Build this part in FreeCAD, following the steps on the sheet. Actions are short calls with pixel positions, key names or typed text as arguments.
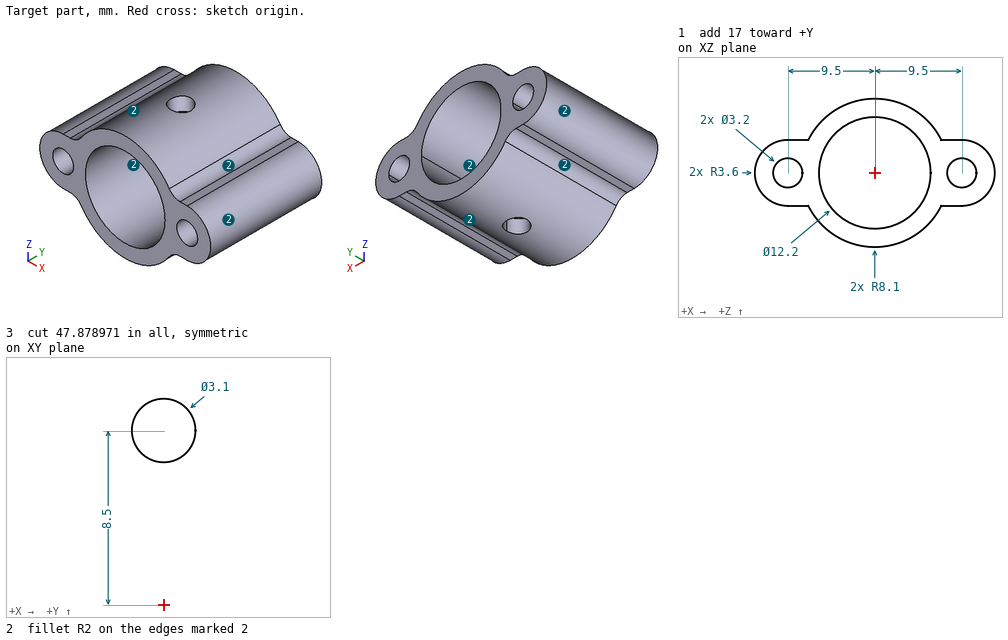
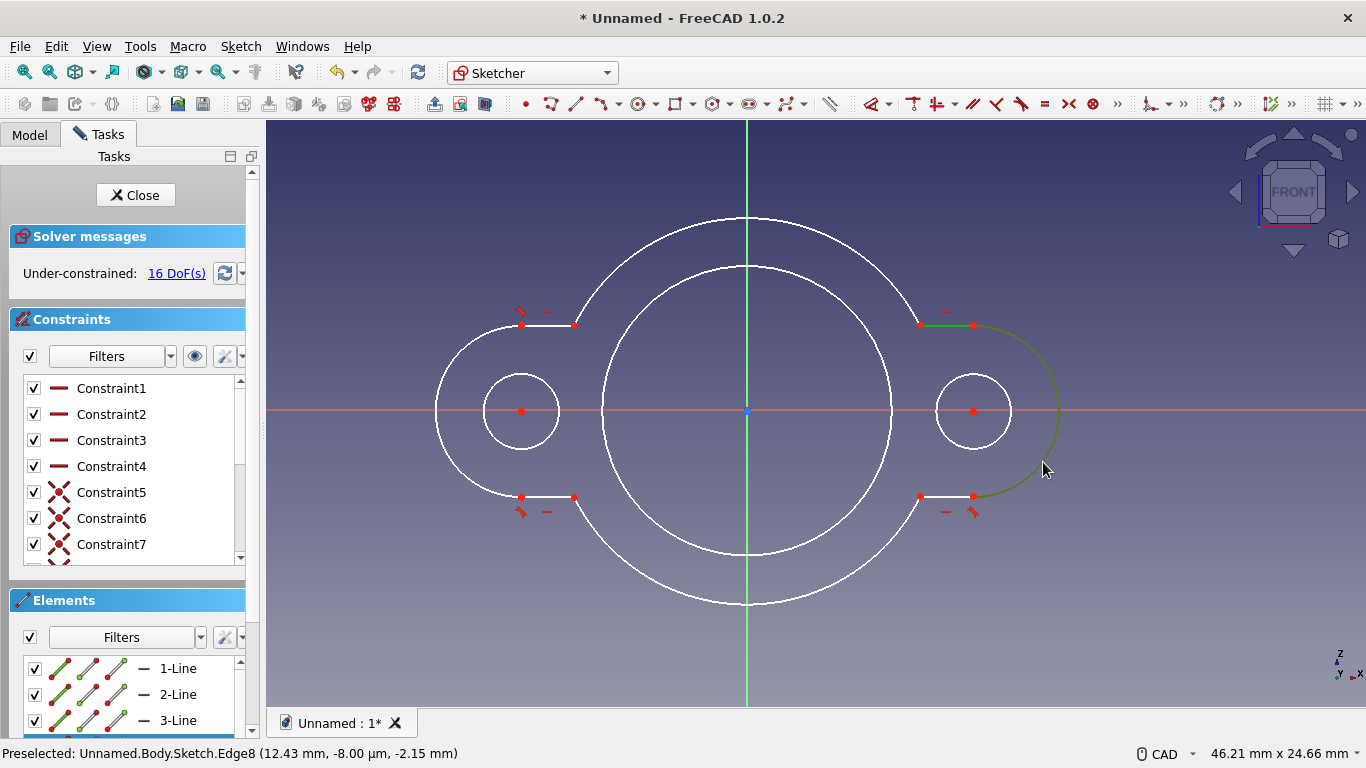
key(t)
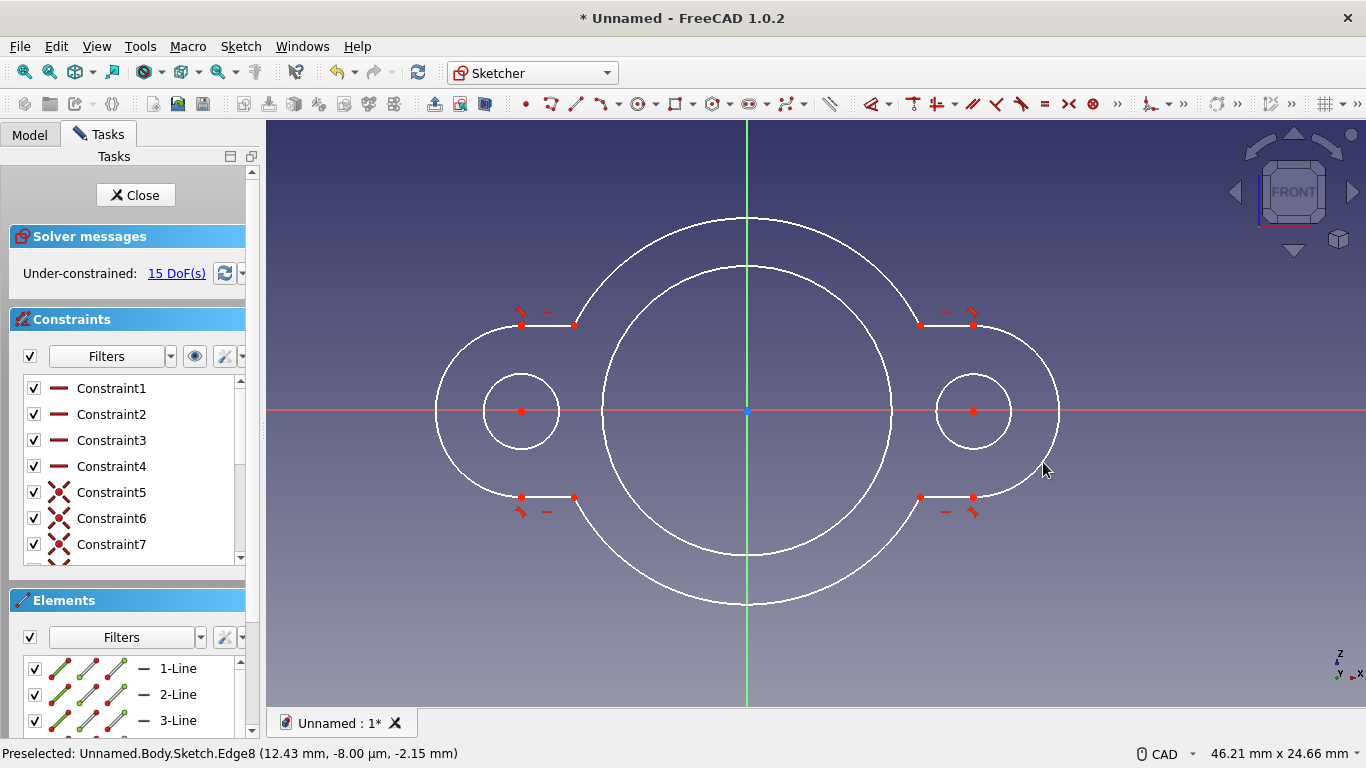
click(849, 308)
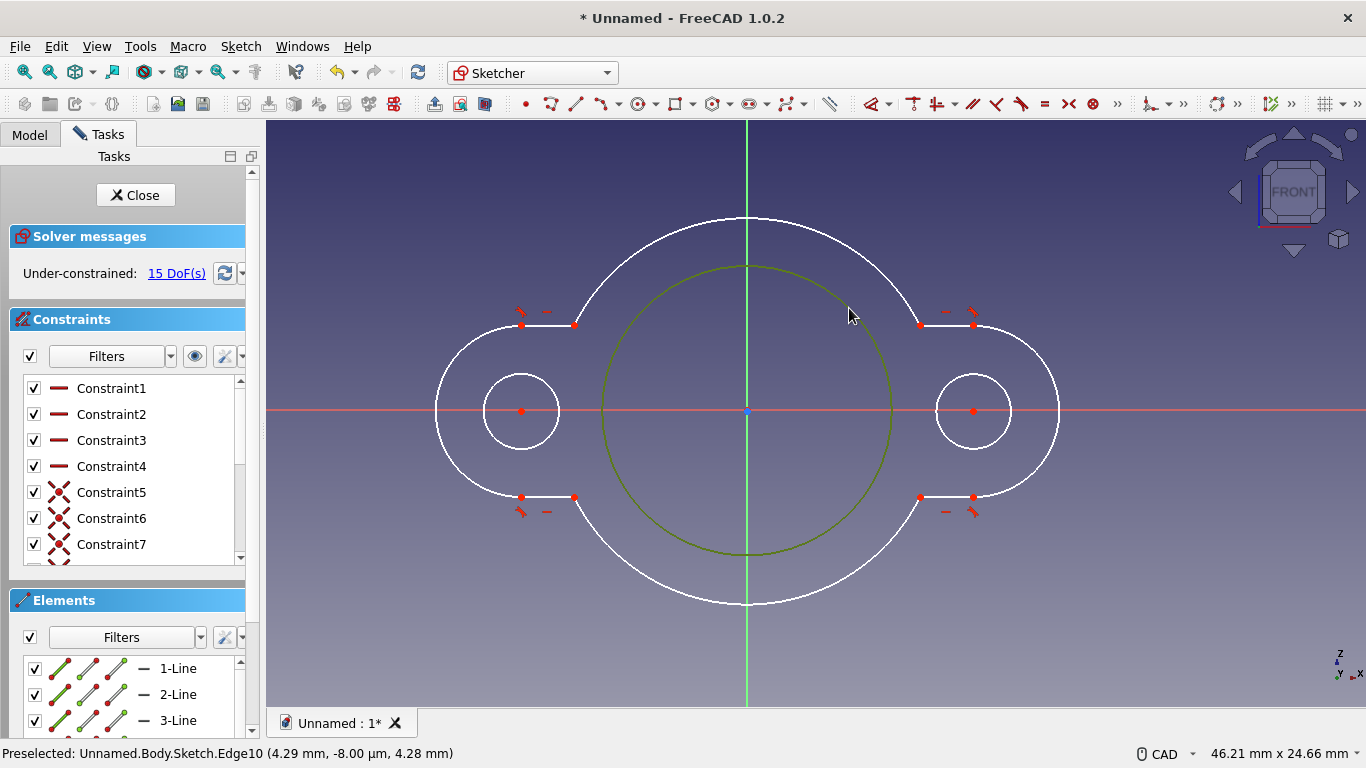
click(664, 586)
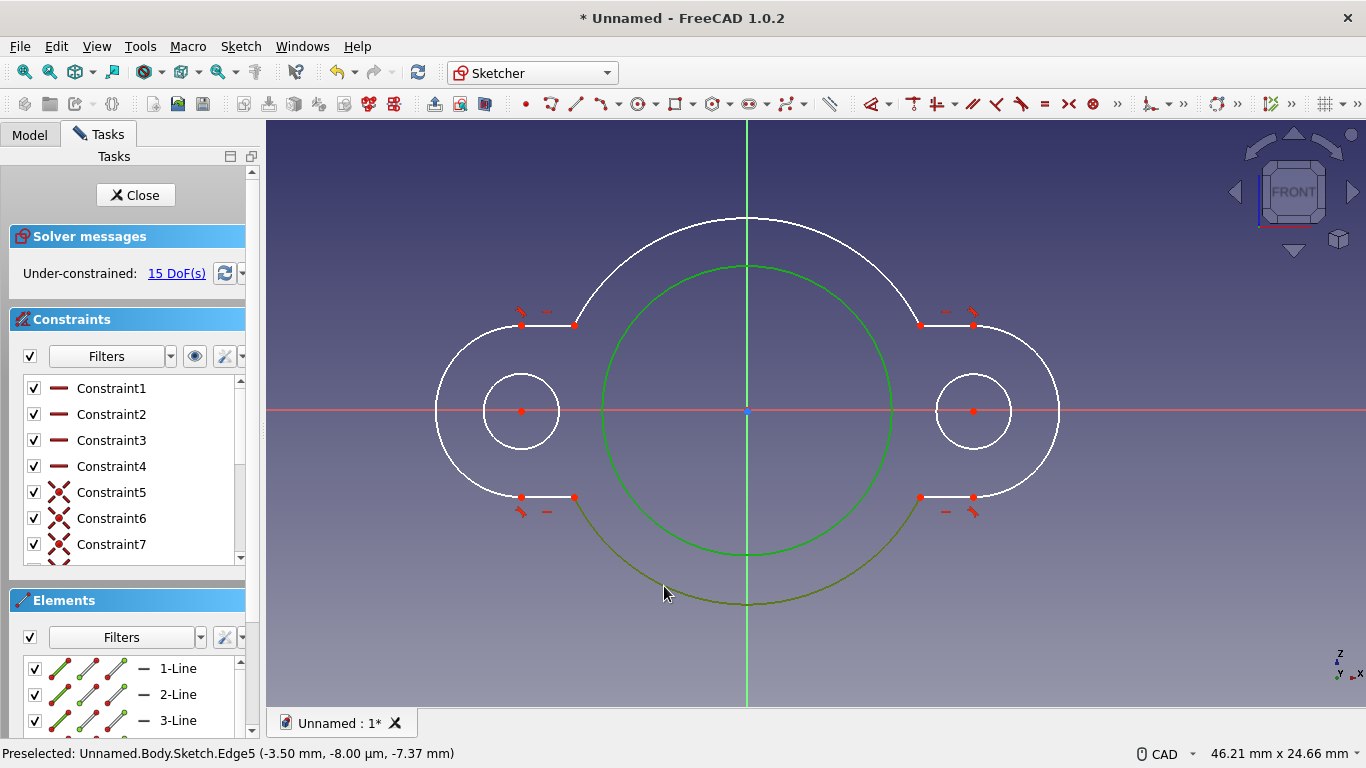
click(913, 104)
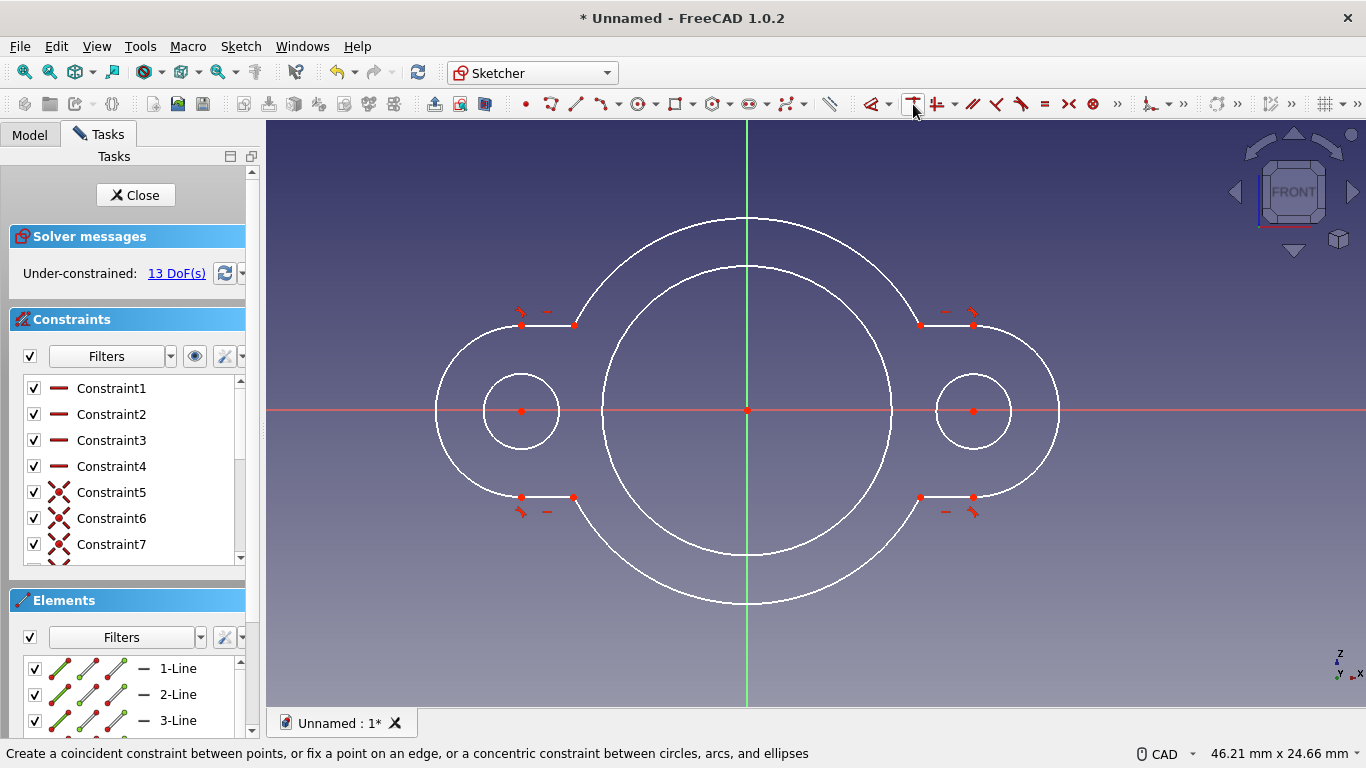
drag(737, 400, 757, 421)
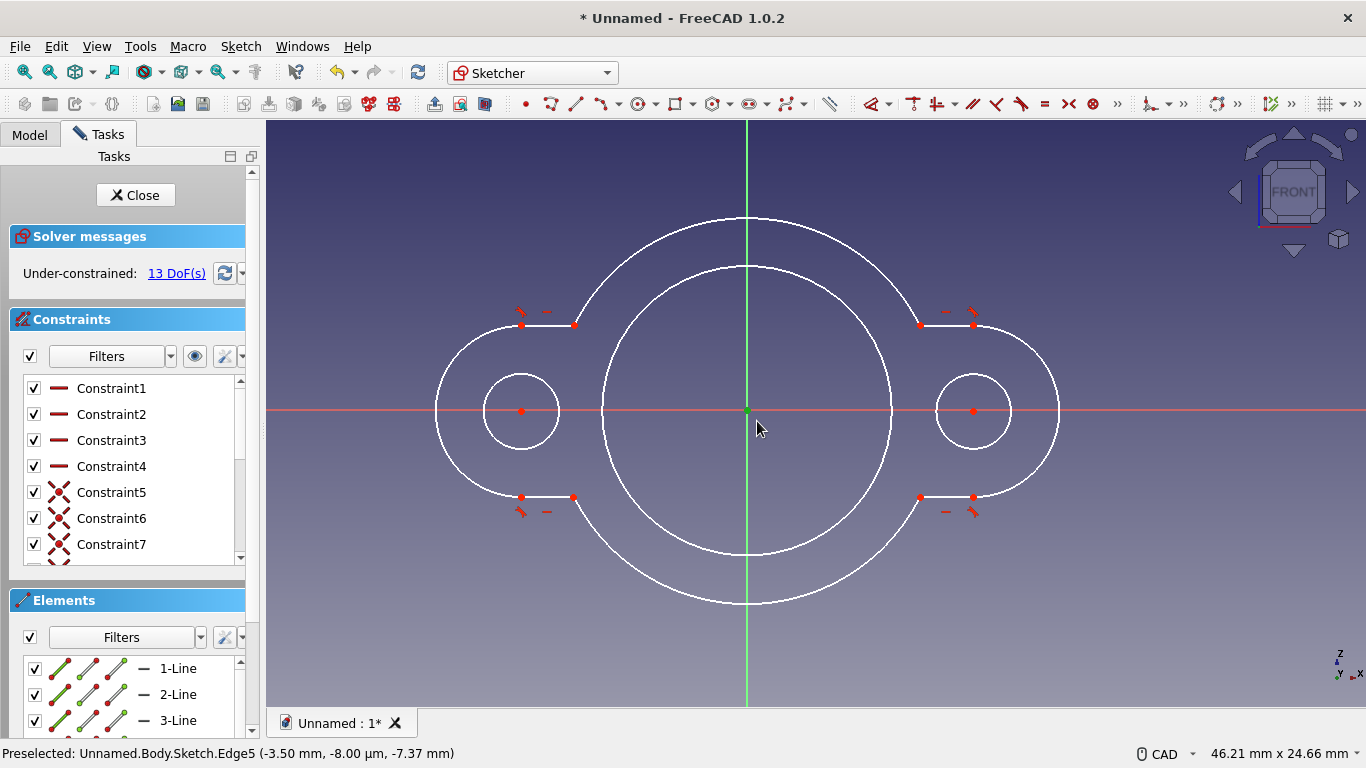
click(913, 104)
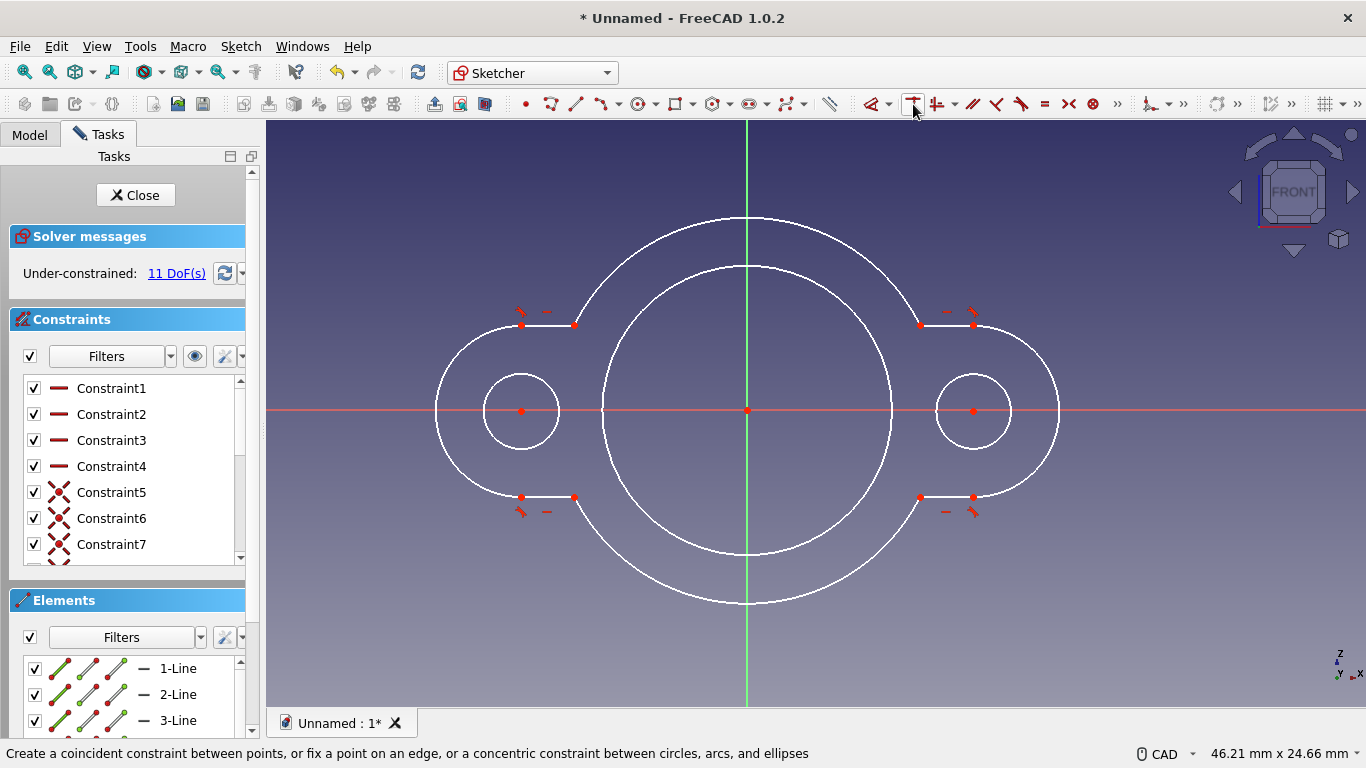
click(664, 585)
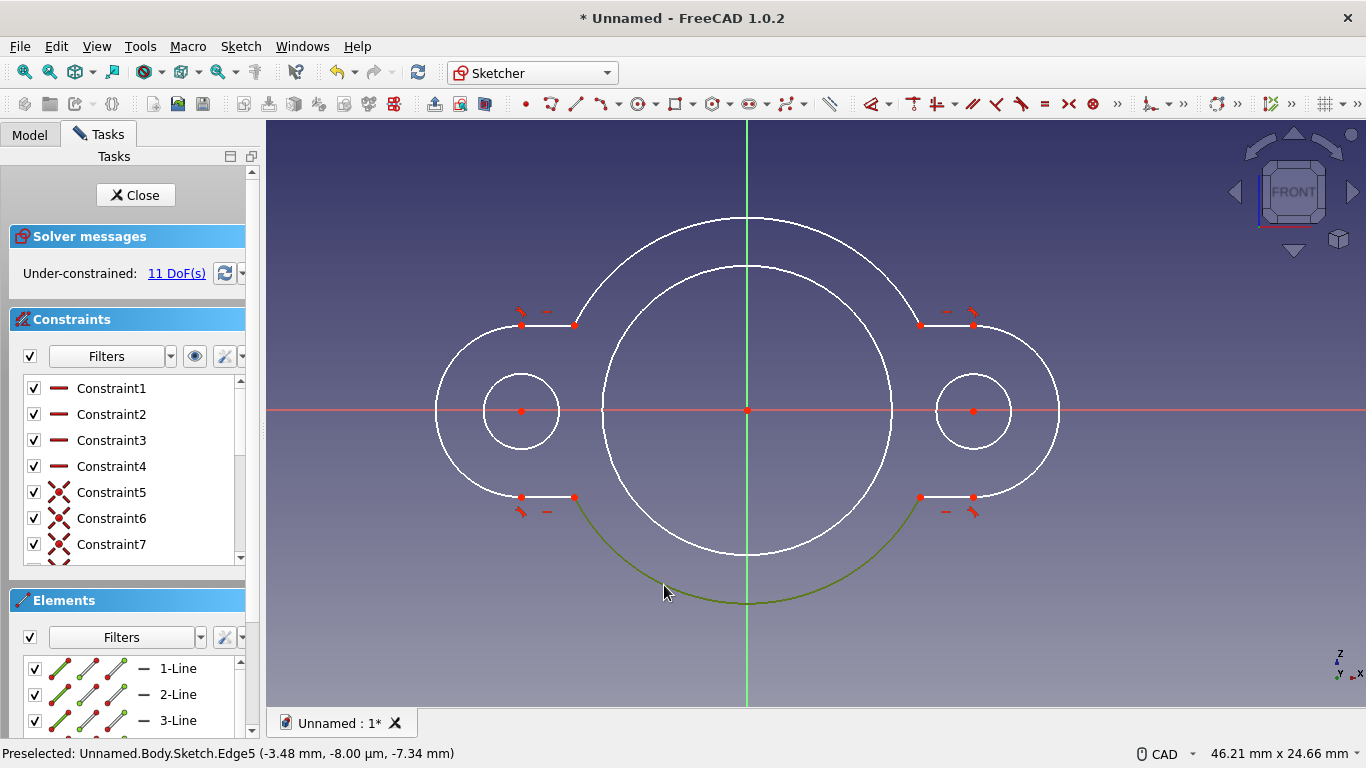
click(830, 237)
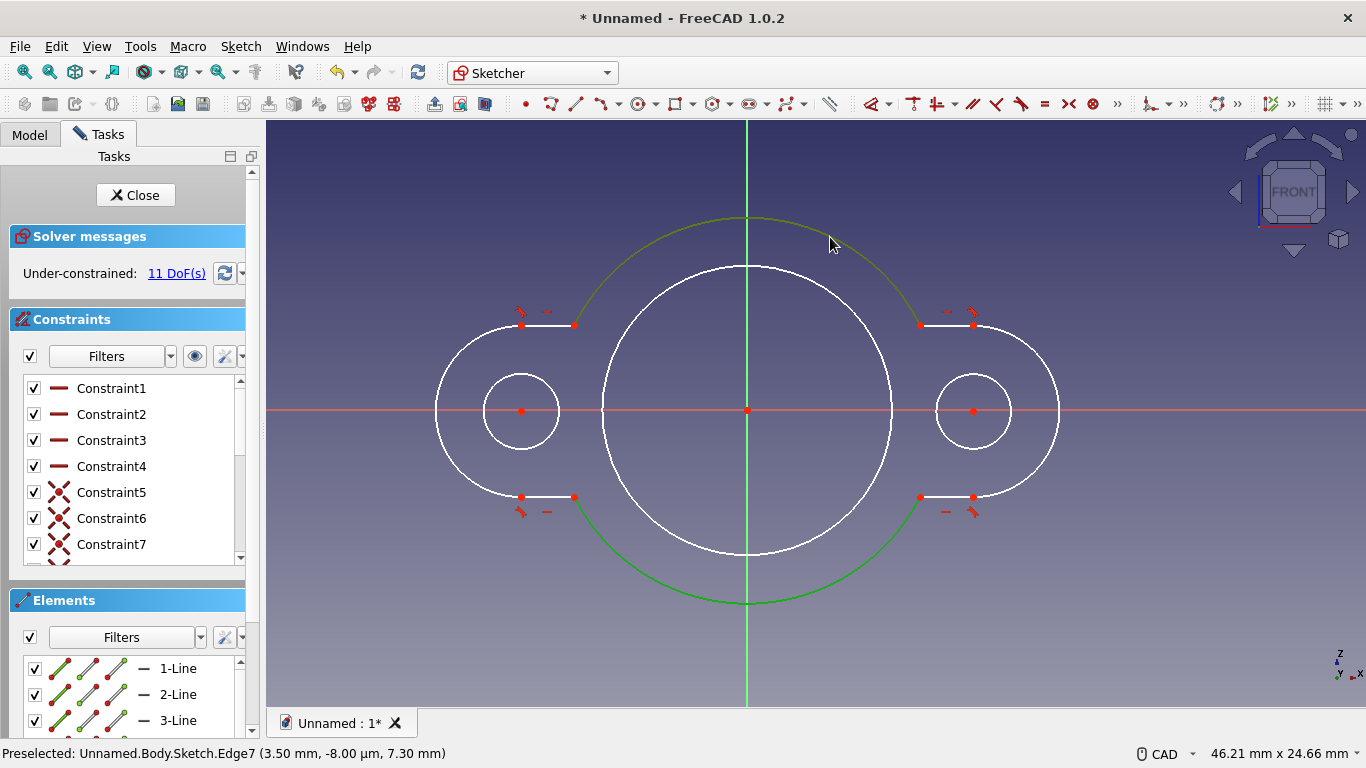
key(e)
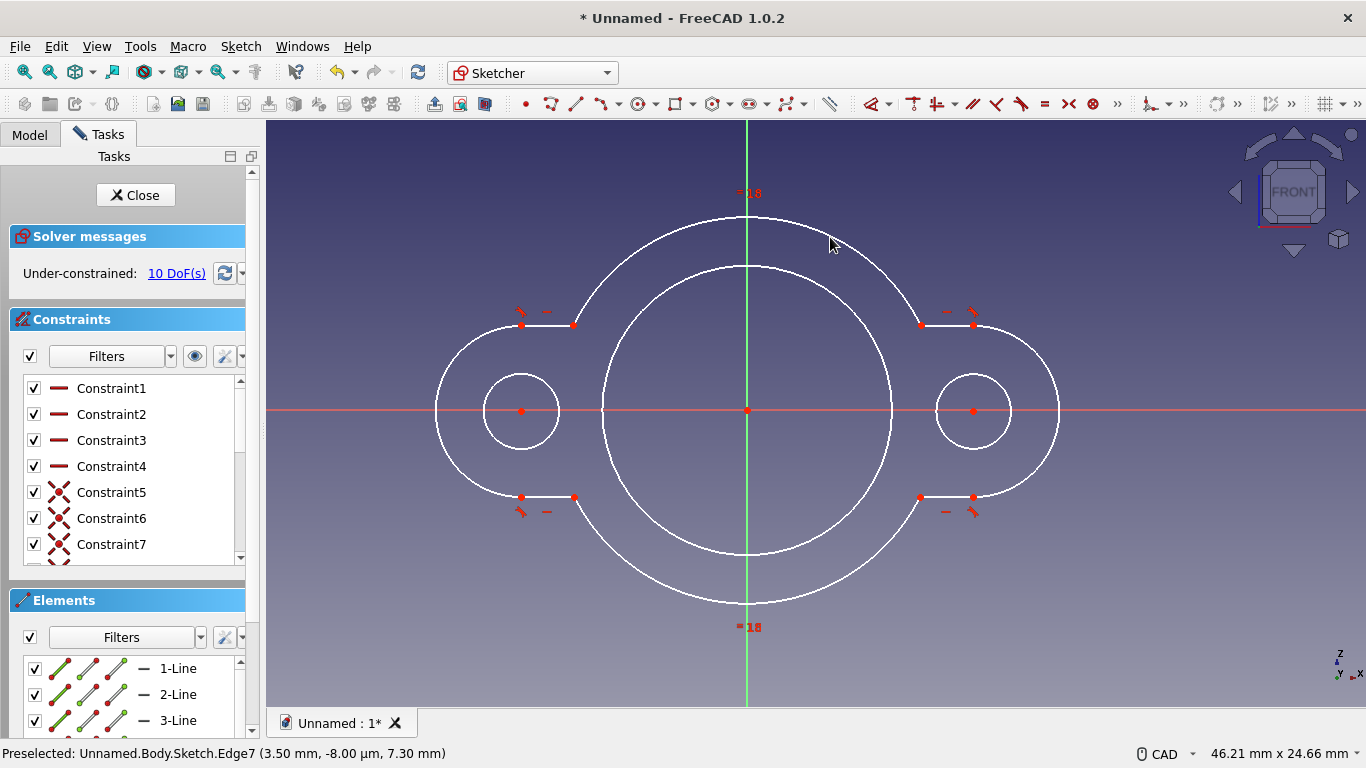
click(452, 361)